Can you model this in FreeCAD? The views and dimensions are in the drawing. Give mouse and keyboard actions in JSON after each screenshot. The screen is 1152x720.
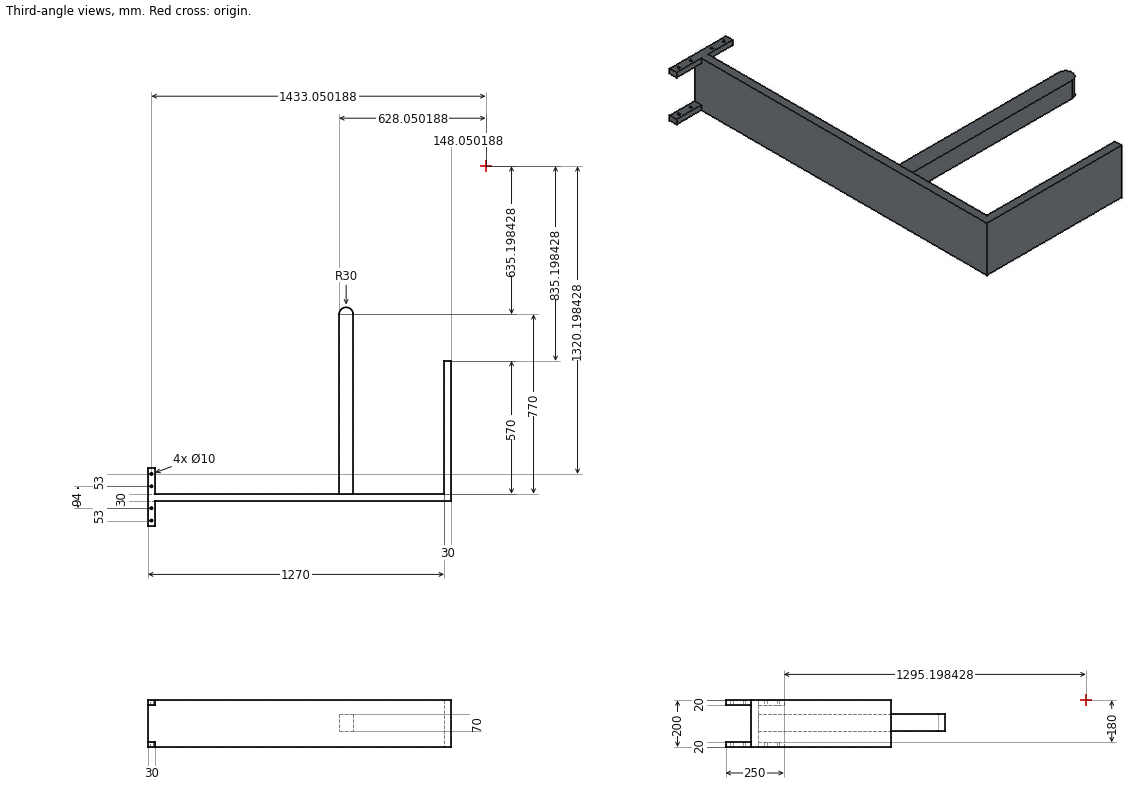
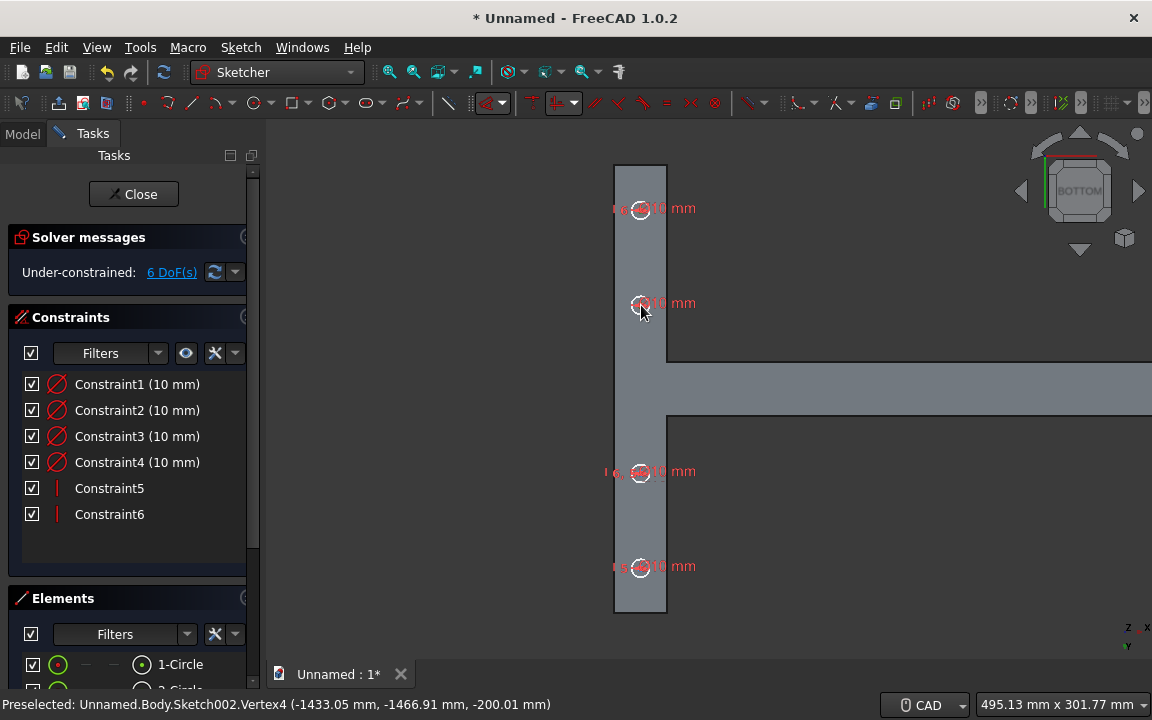
{"action": "key", "text": "v"}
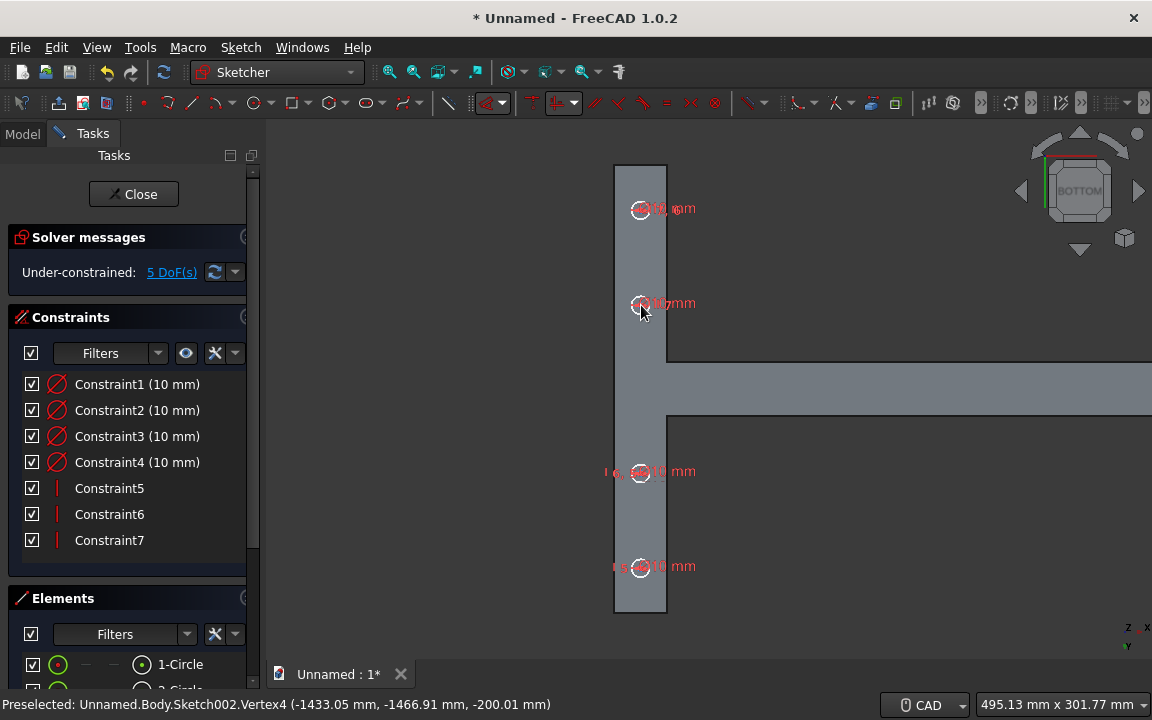
{"action": "left_click", "coordinate": [641, 568]}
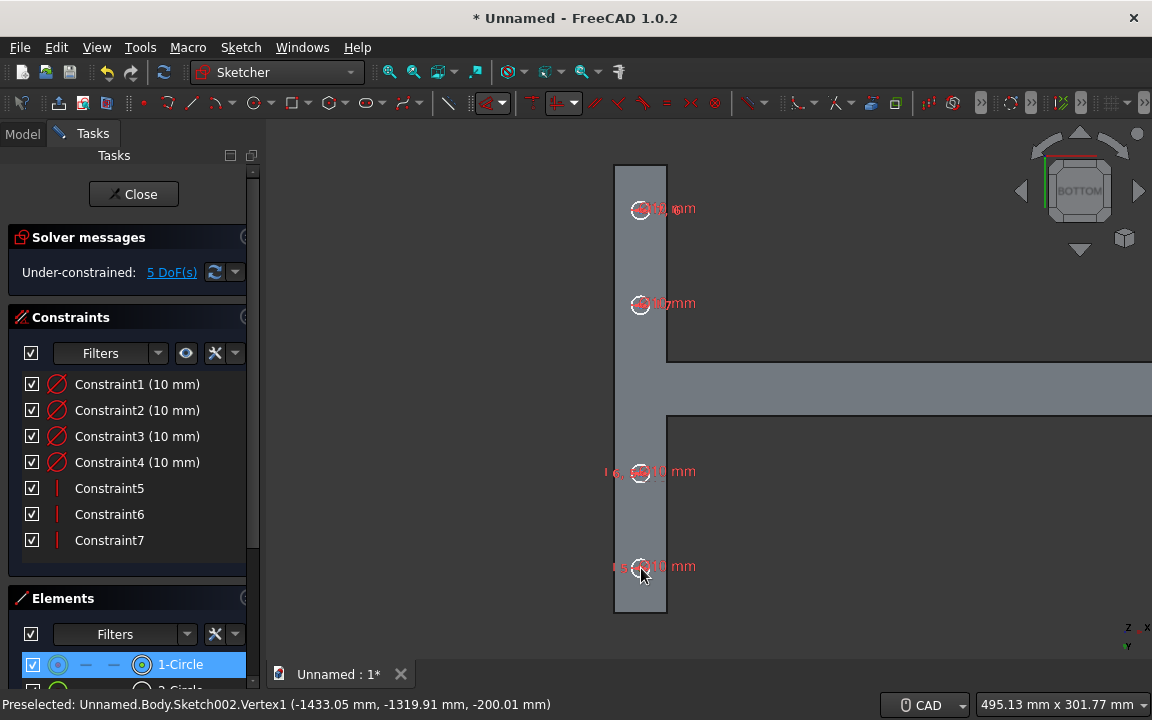
{"action": "left_click", "coordinate": [641, 474]}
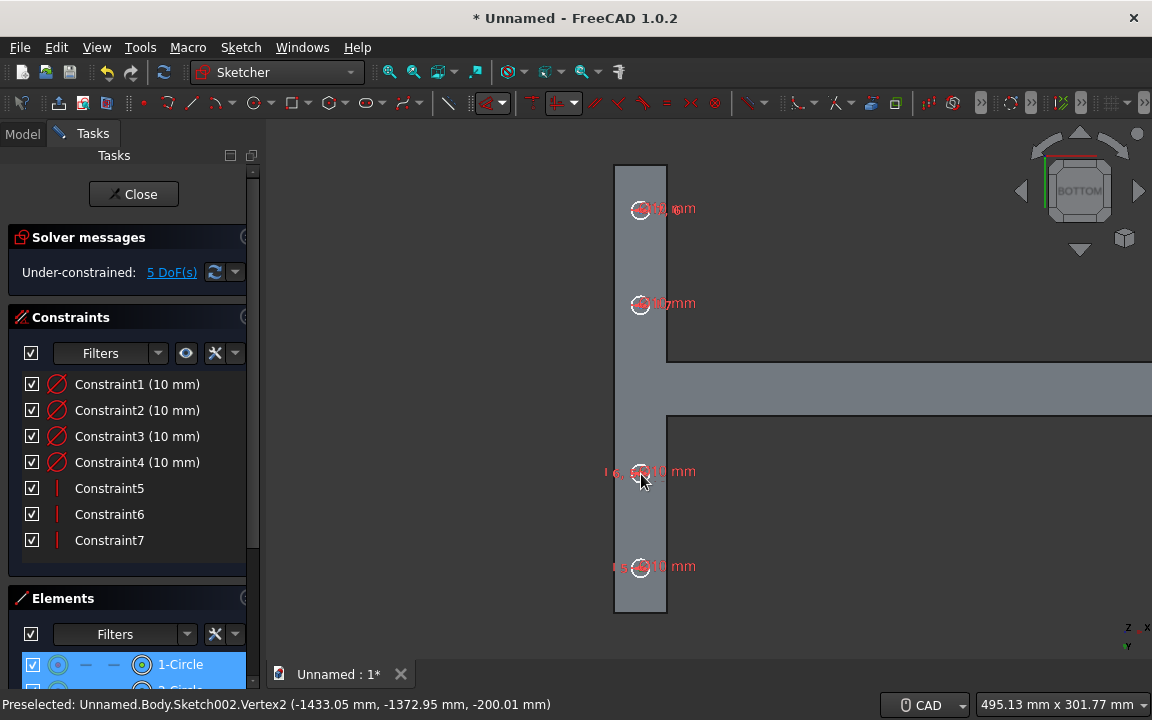
{"action": "left_click", "coordinate": [504, 104]}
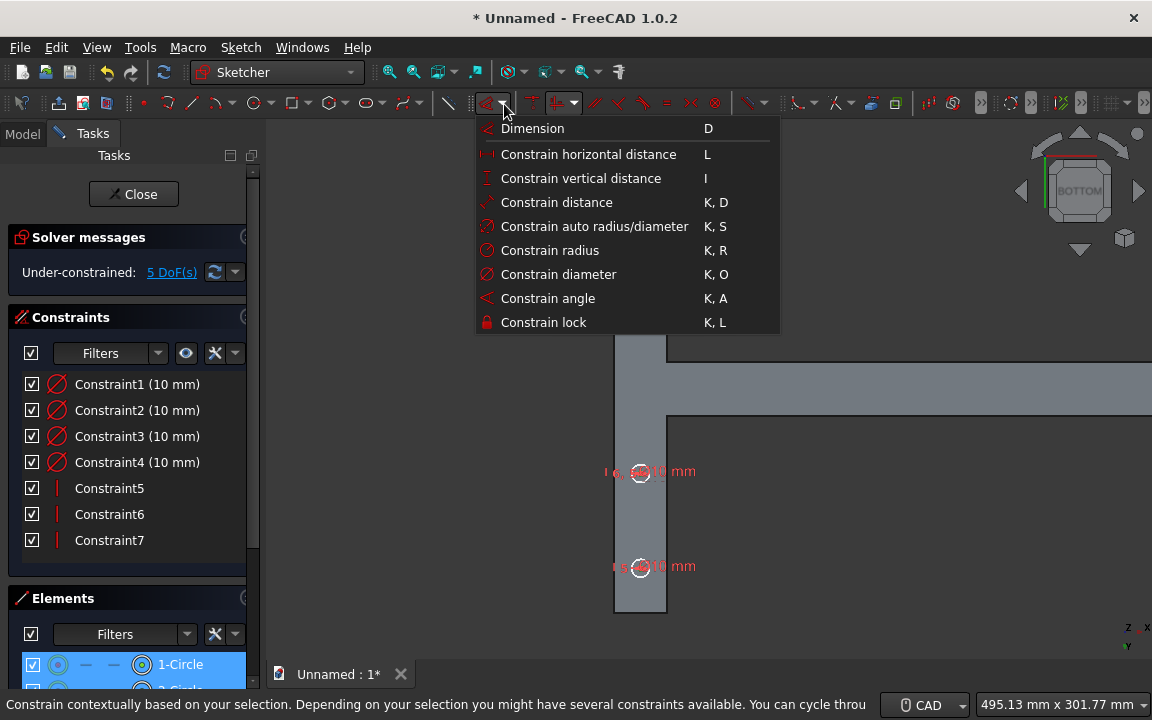
{"action": "left_click", "coordinate": [628, 178]}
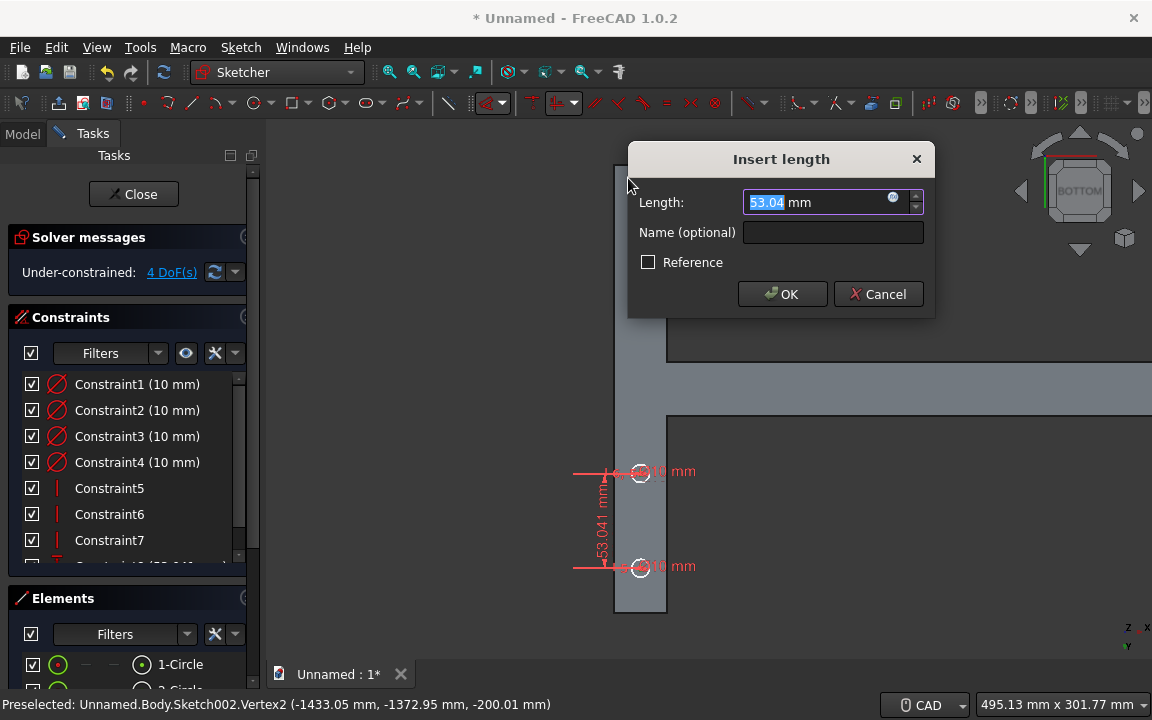
{"action": "type", "text": "53"}
{"action": "key", "text": "Return"}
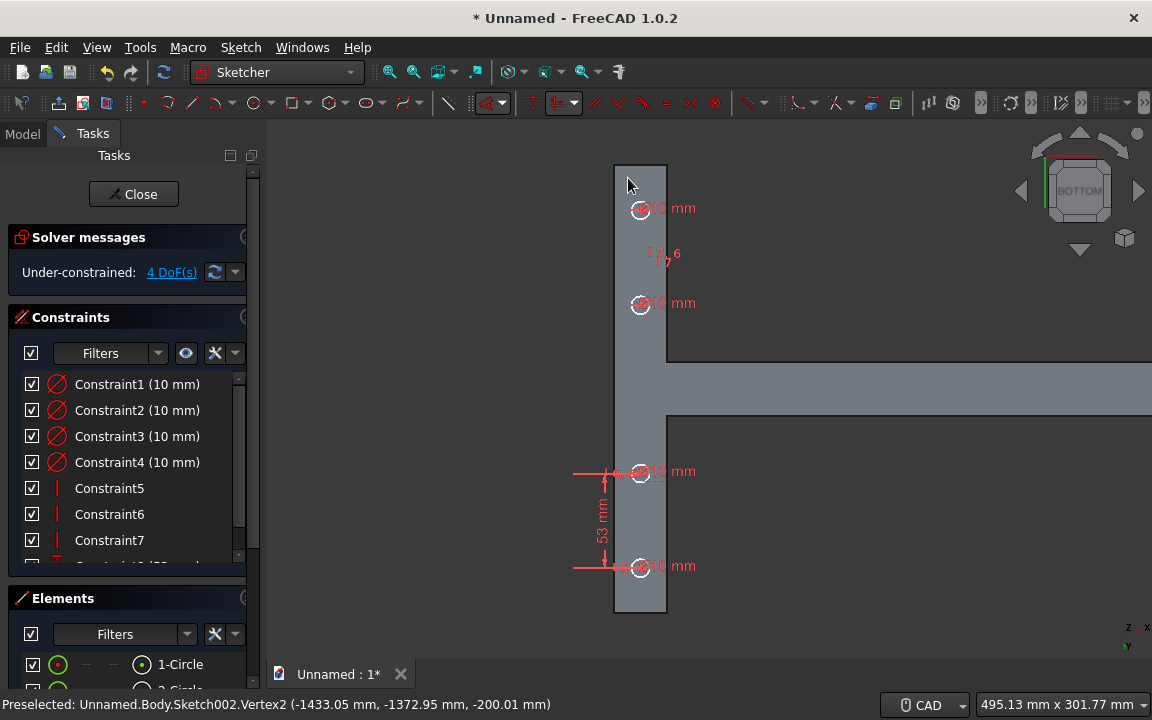
{"action": "left_click", "coordinate": [641, 210]}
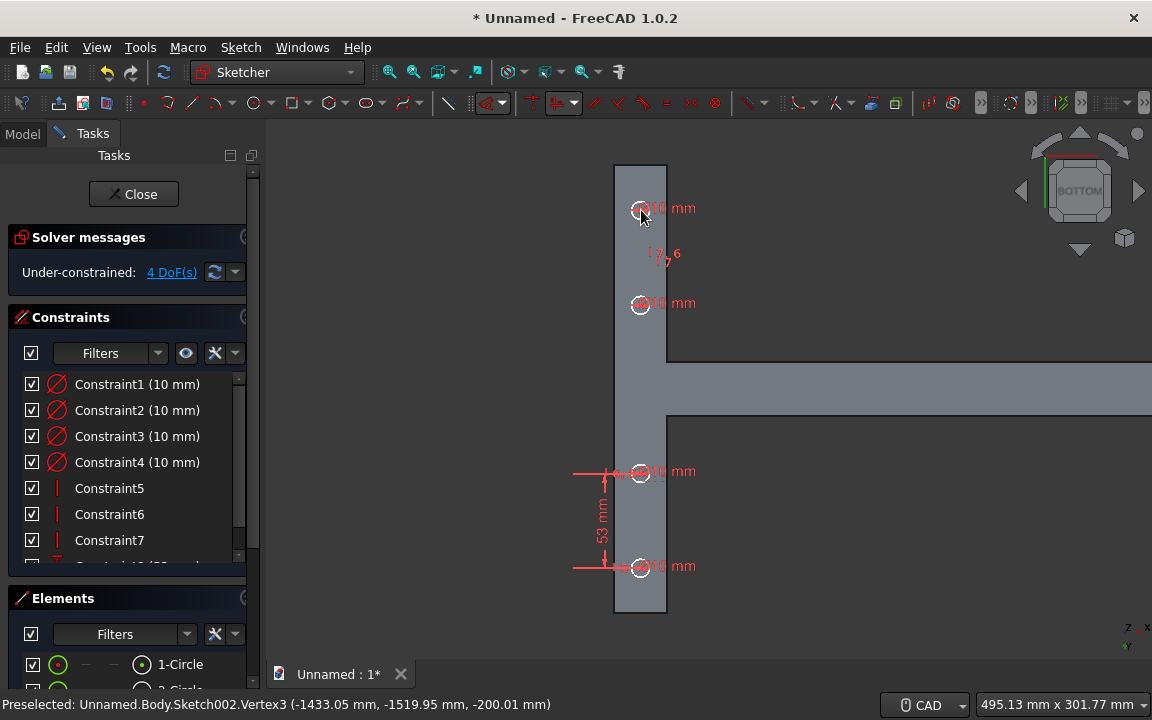
{"action": "left_click", "coordinate": [641, 305]}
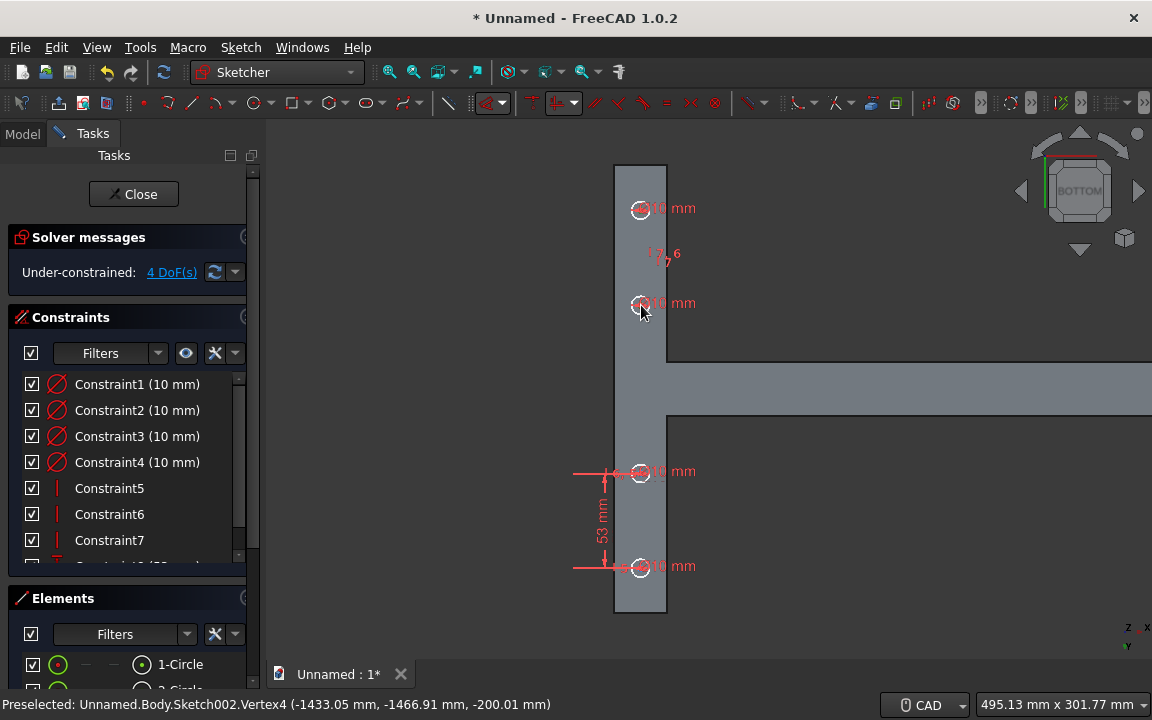
{"action": "key", "text": "i"}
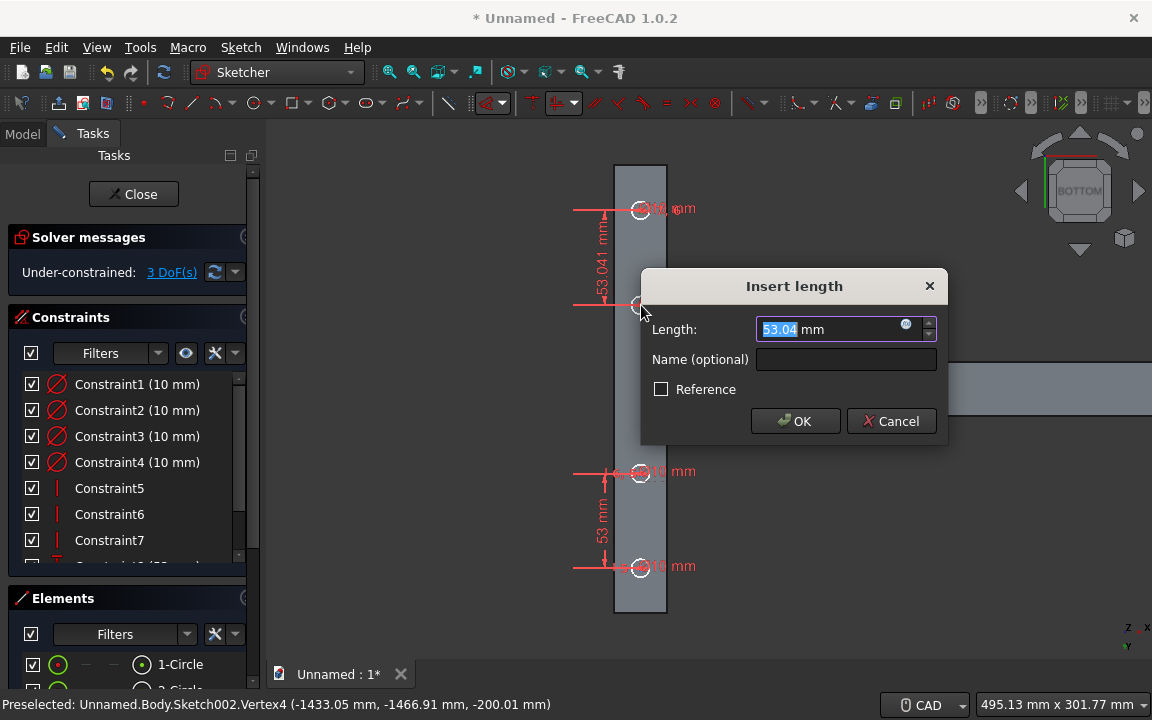
{"action": "type", "text": "53"}
{"action": "key", "text": "Return"}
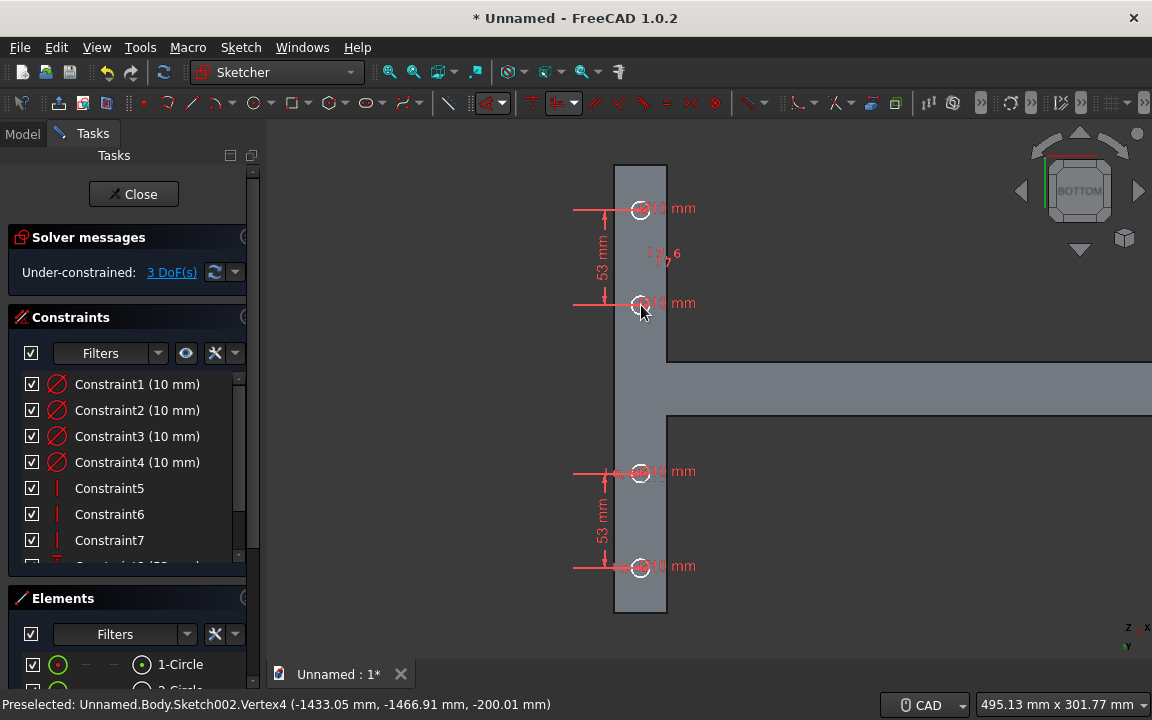
{"action": "left_click", "coordinate": [641, 474]}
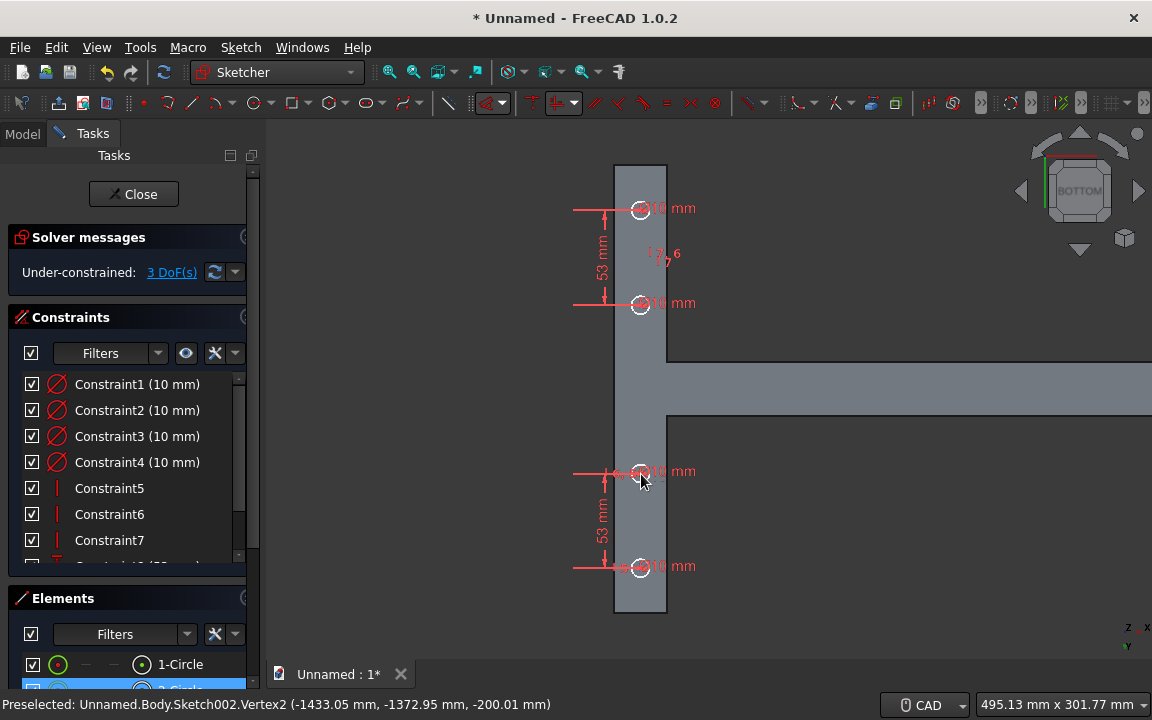
{"action": "left_click", "coordinate": [641, 305]}